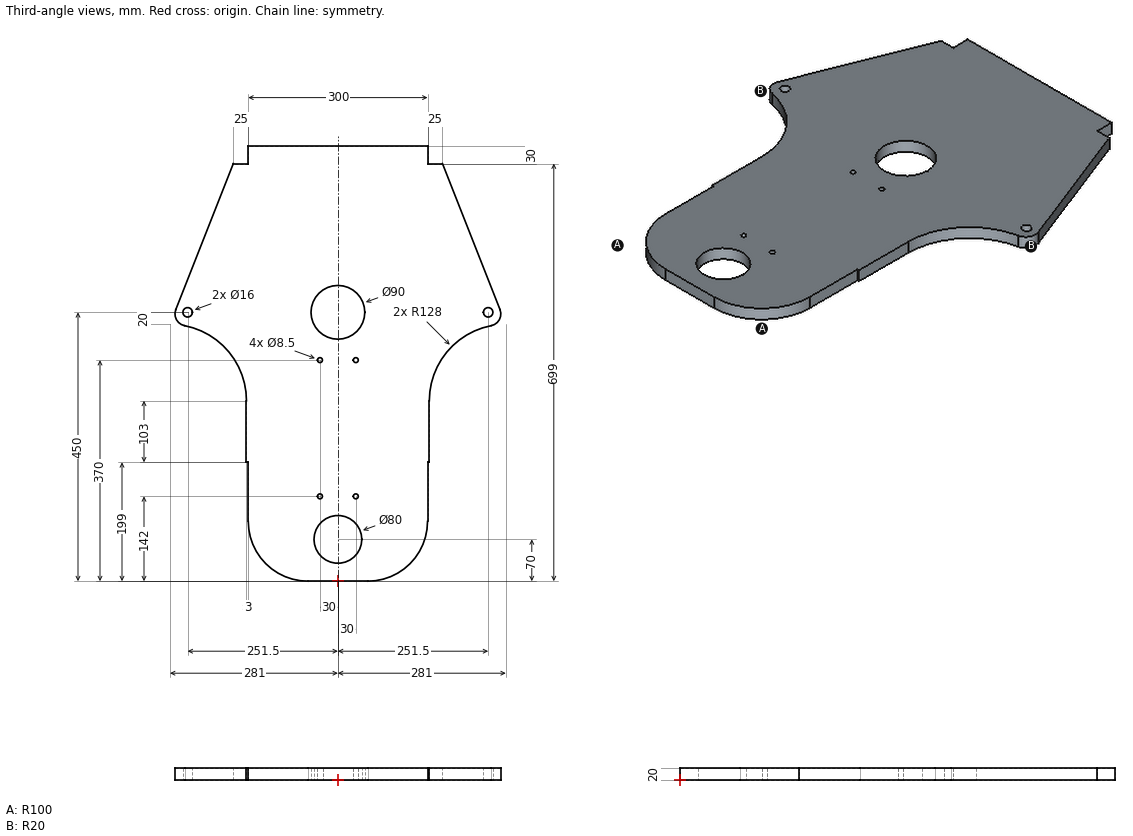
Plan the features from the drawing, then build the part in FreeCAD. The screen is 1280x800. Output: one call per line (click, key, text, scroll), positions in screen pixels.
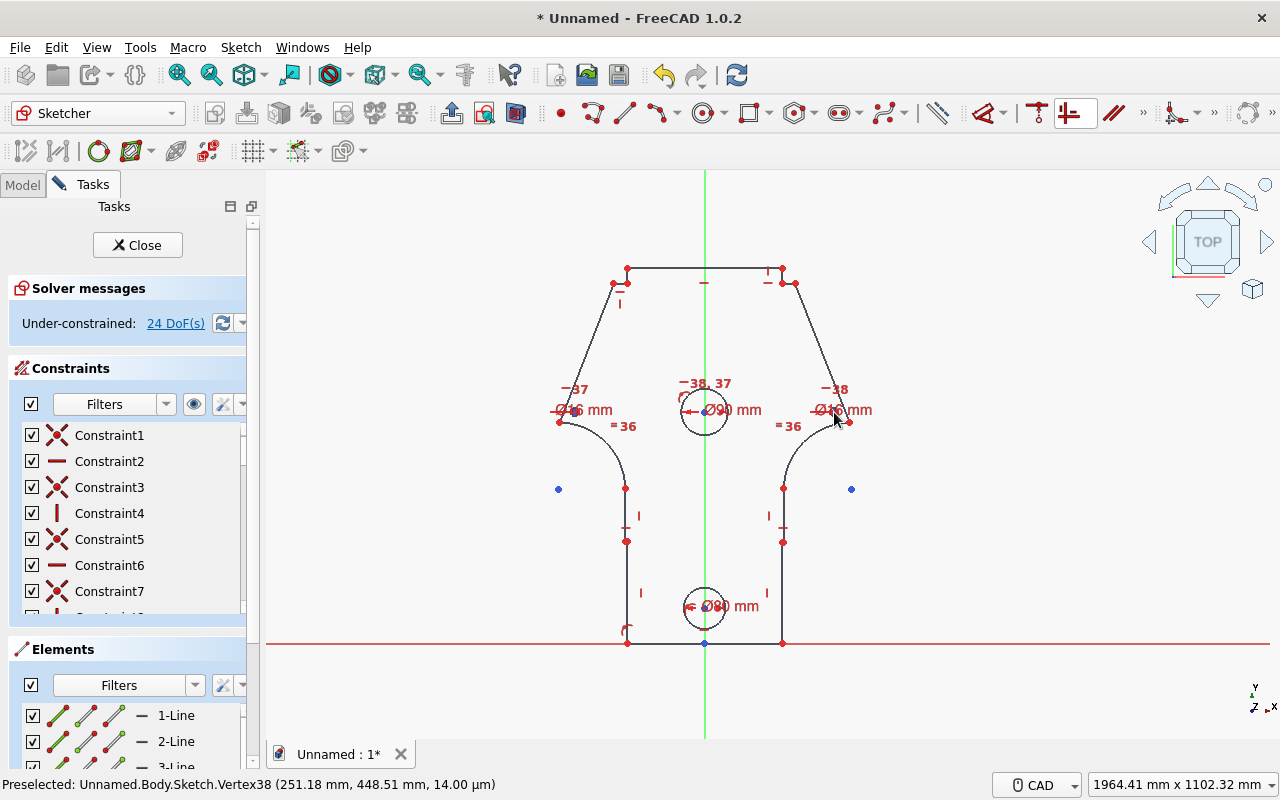
click(558, 490)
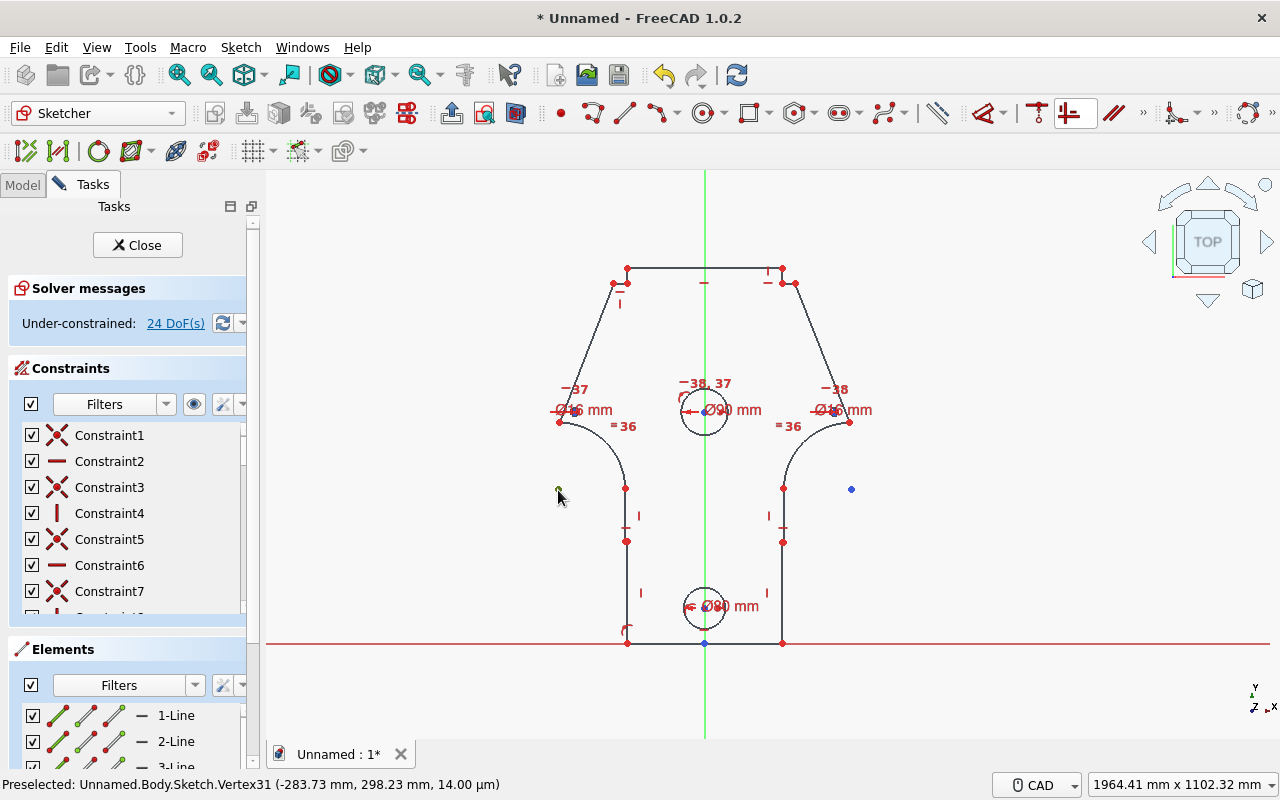
click(851, 490)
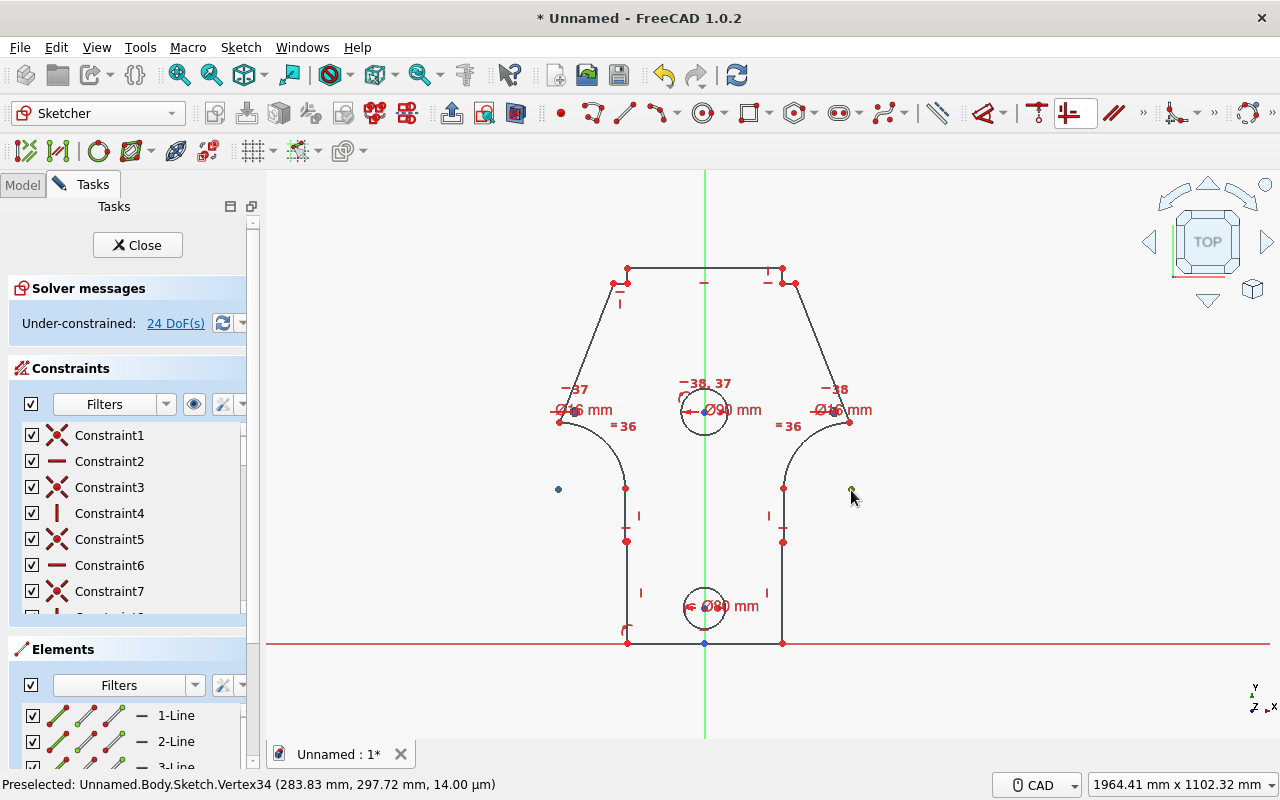
click(705, 674)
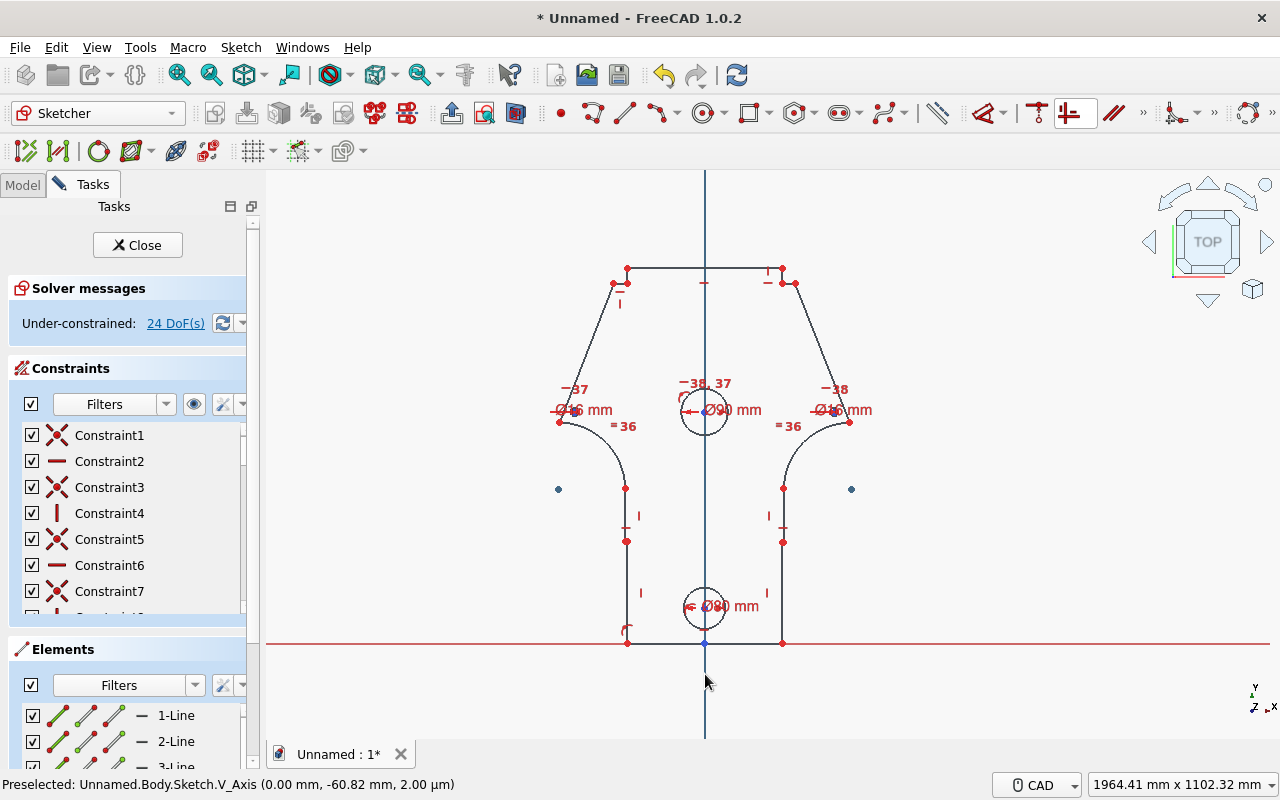
key(s)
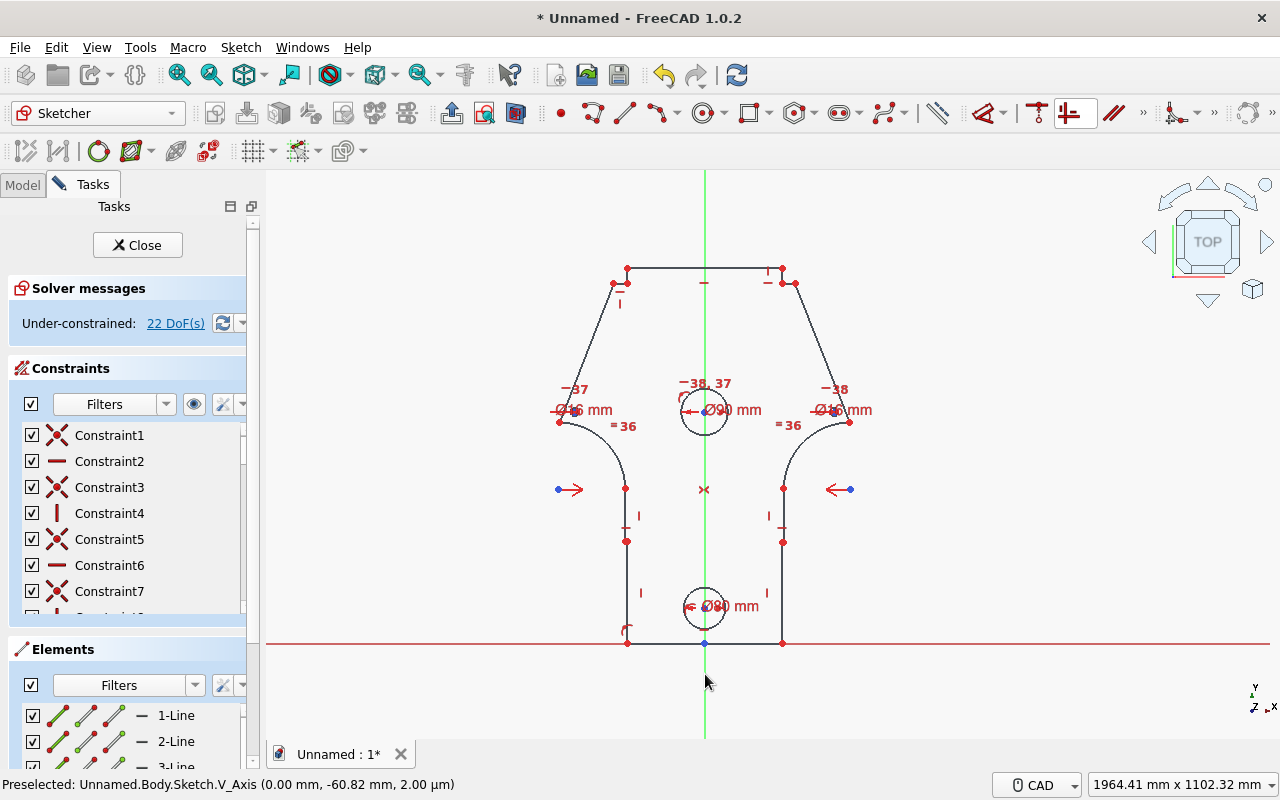
click(782, 284)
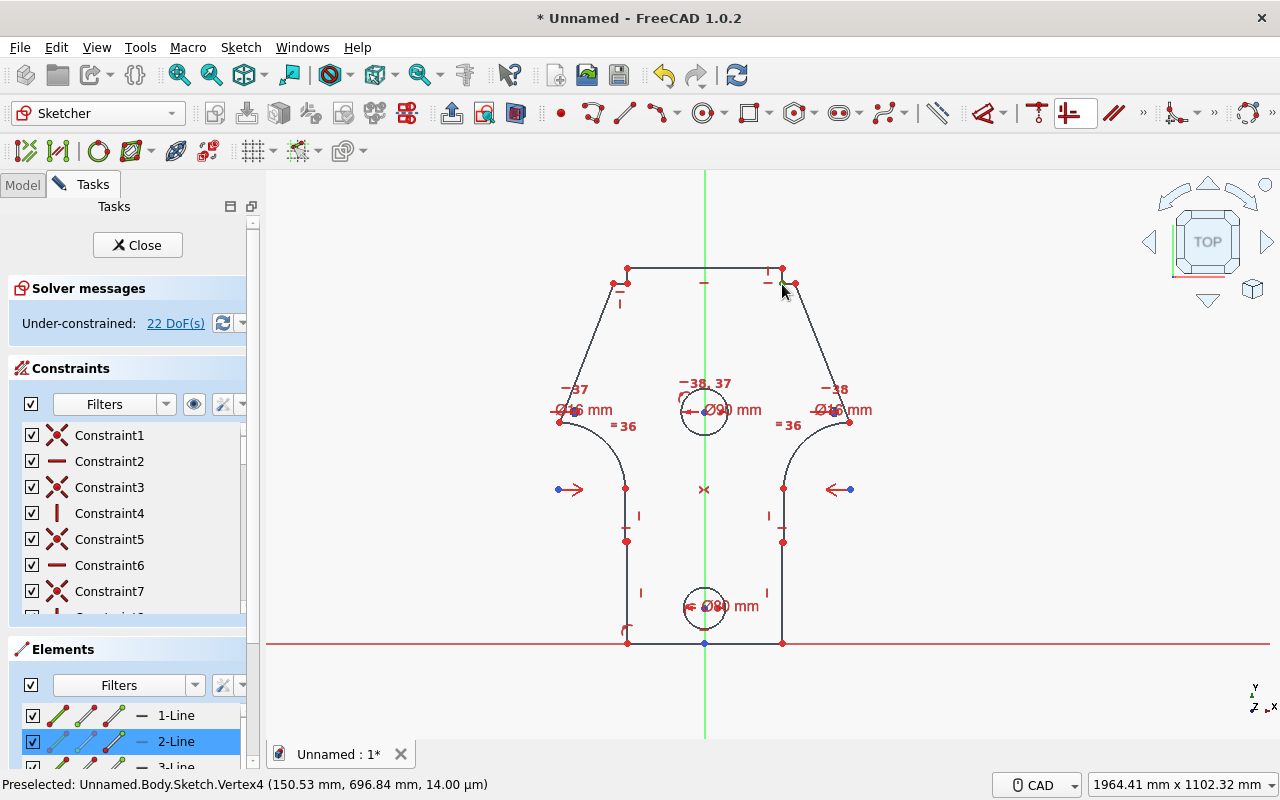
click(627, 284)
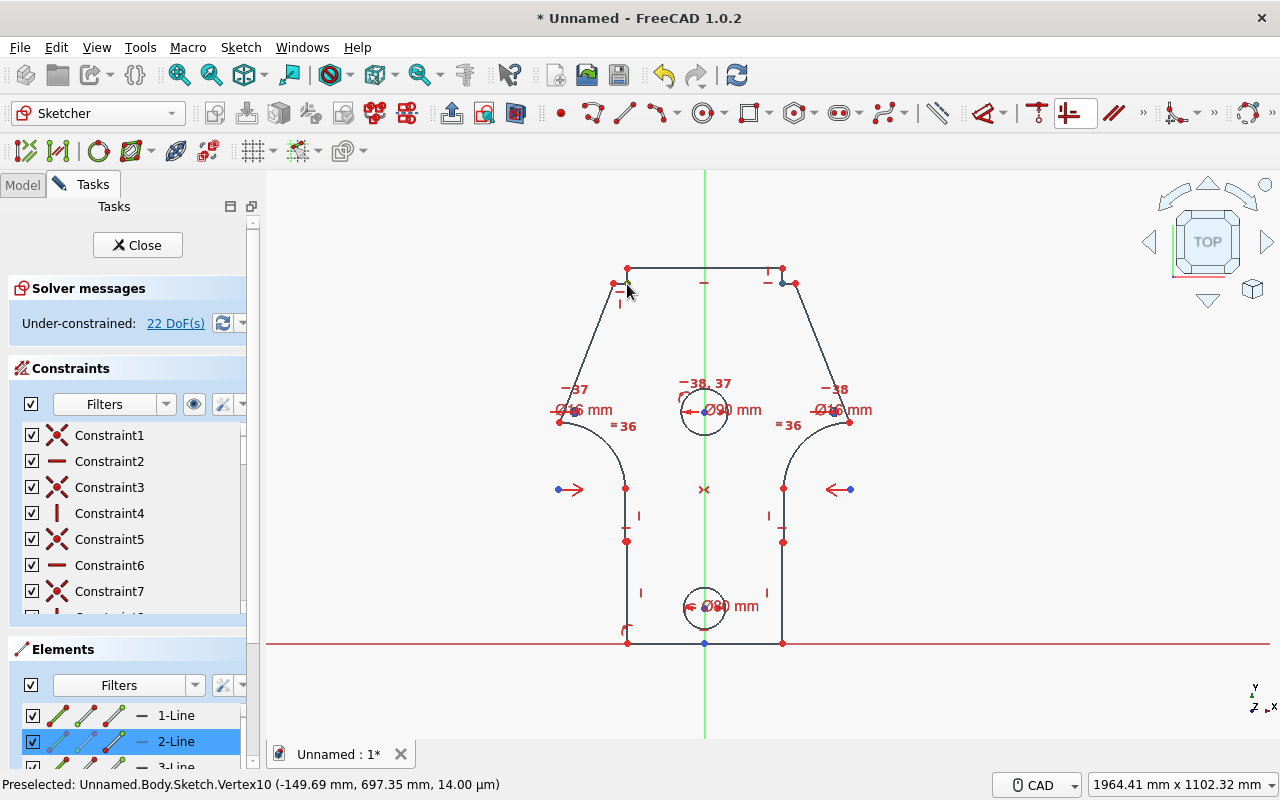
click(705, 674)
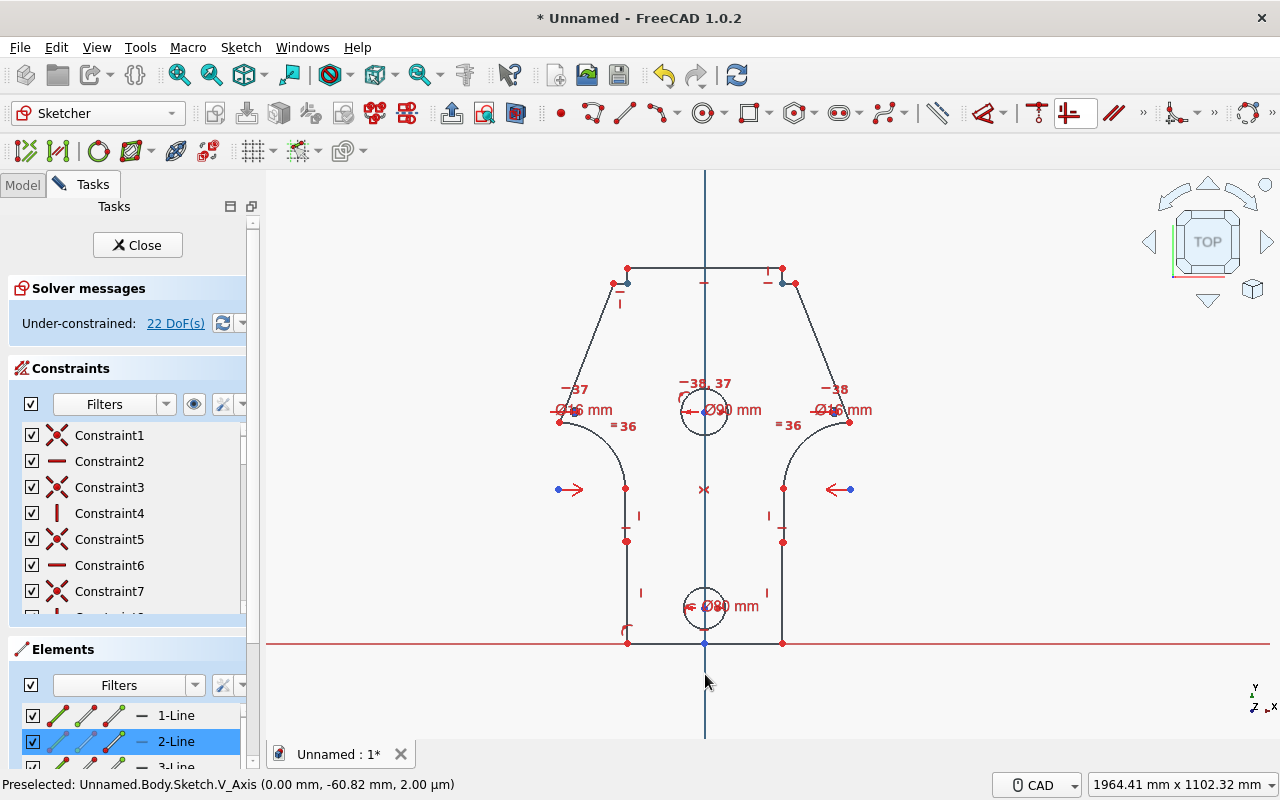
key(s)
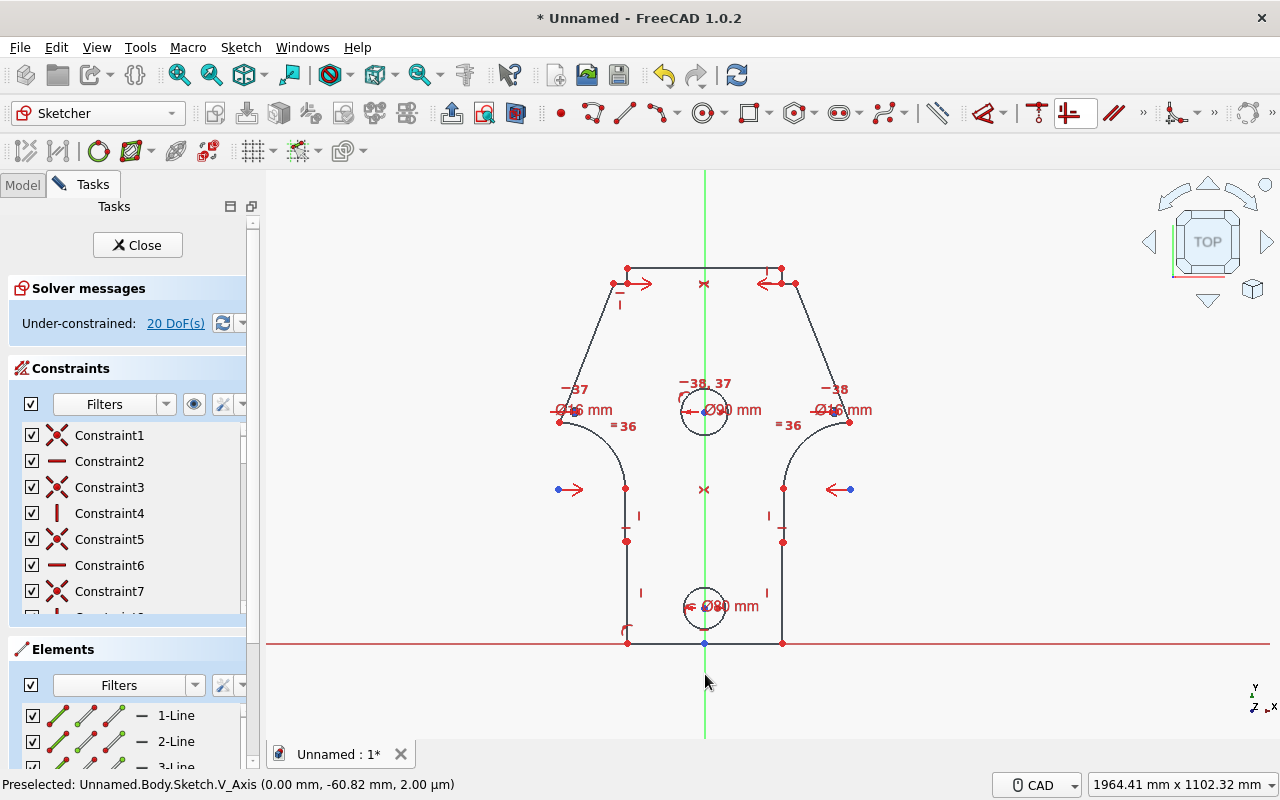
scroll(627, 541, up, 10)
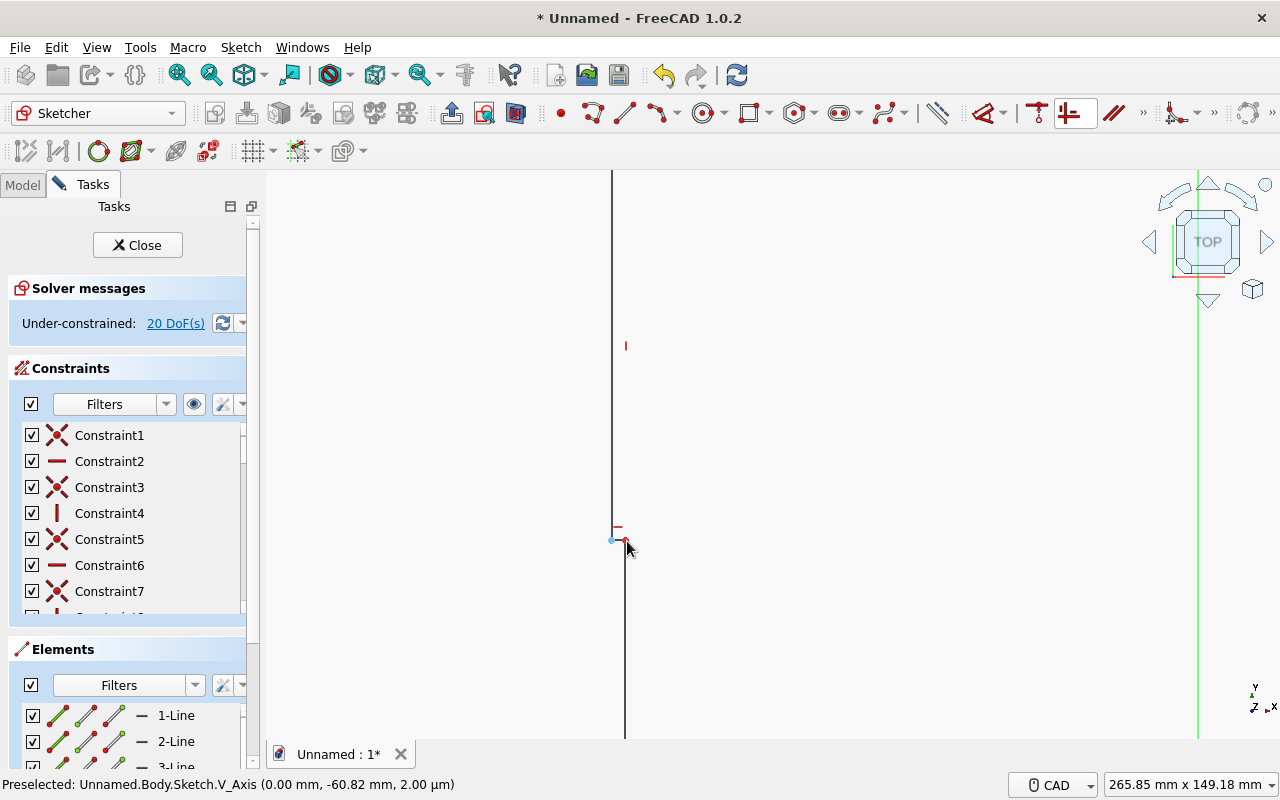
click(625, 540)